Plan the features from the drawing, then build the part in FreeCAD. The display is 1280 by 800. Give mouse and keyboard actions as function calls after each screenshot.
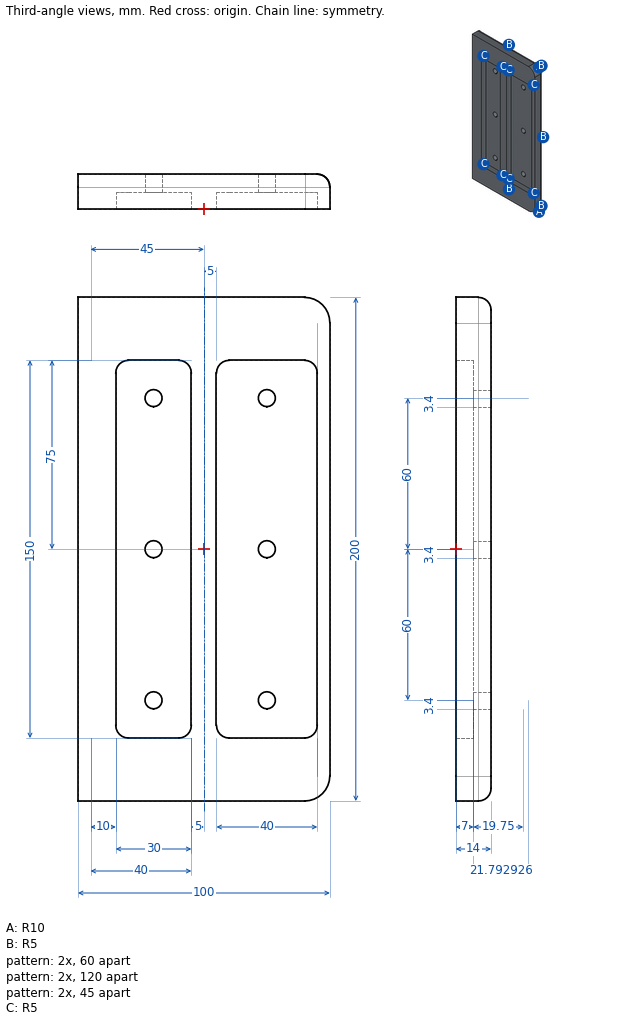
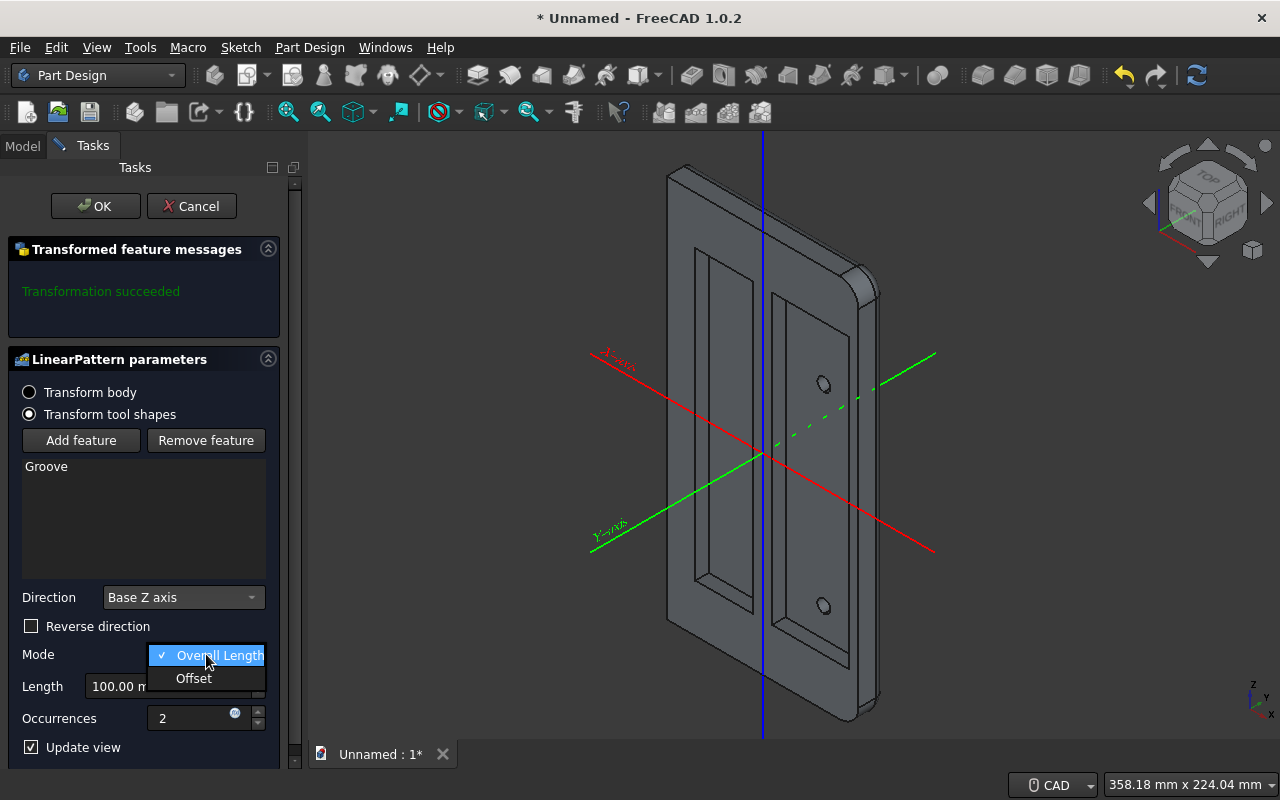
click(206, 678)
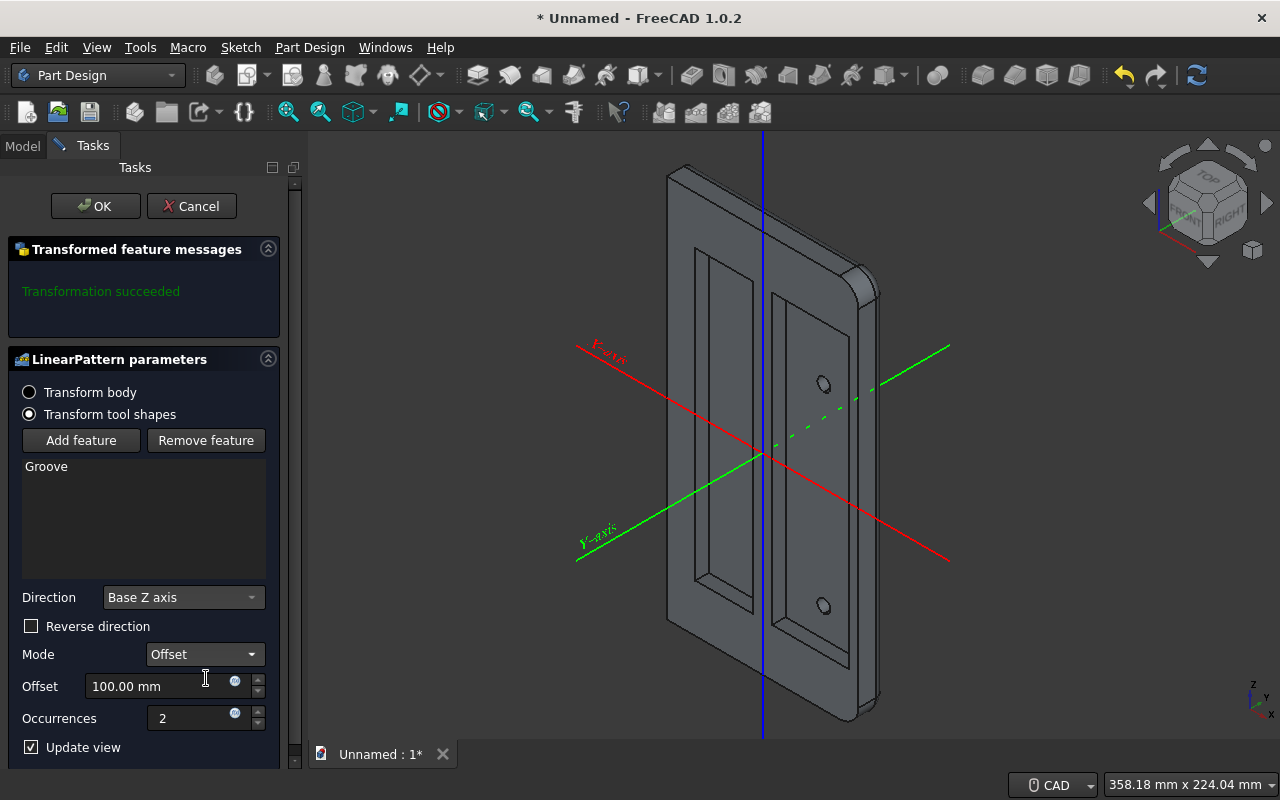
triple_click(168, 686)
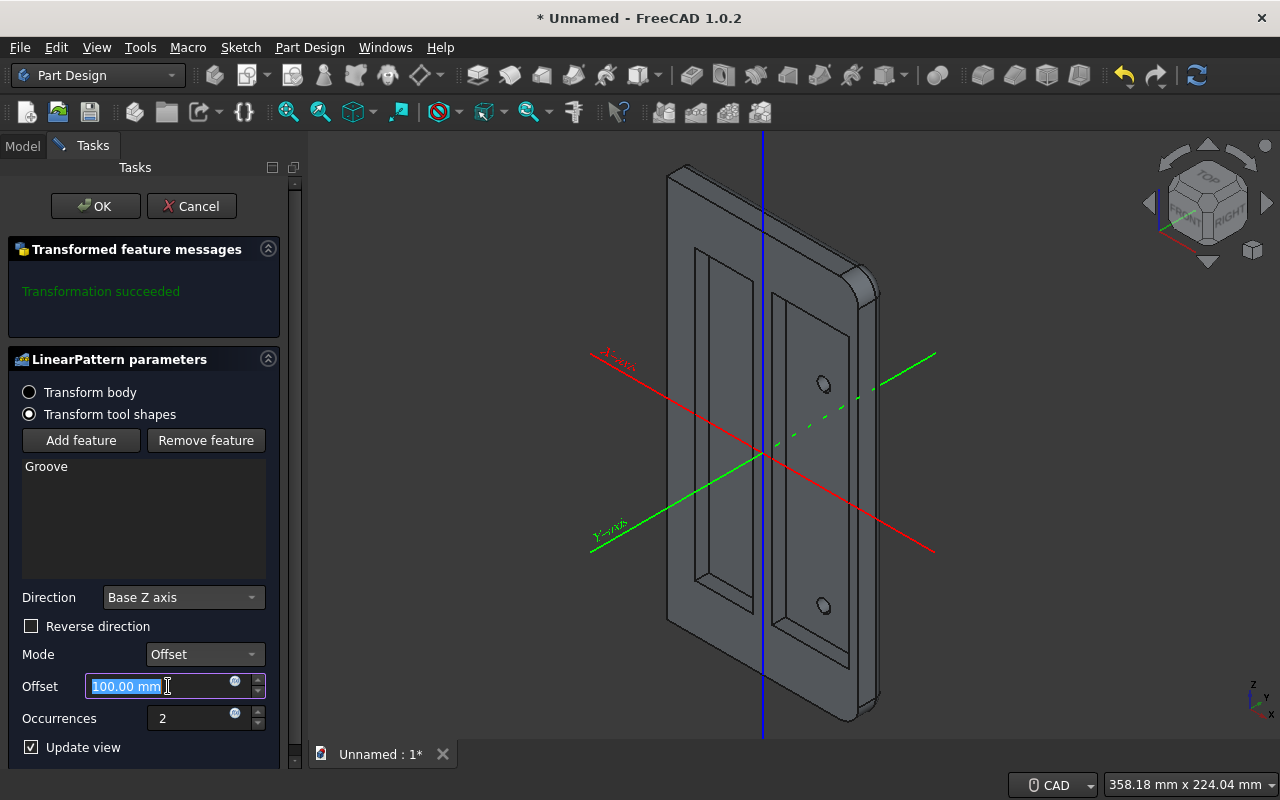
text(60)
key(Tab)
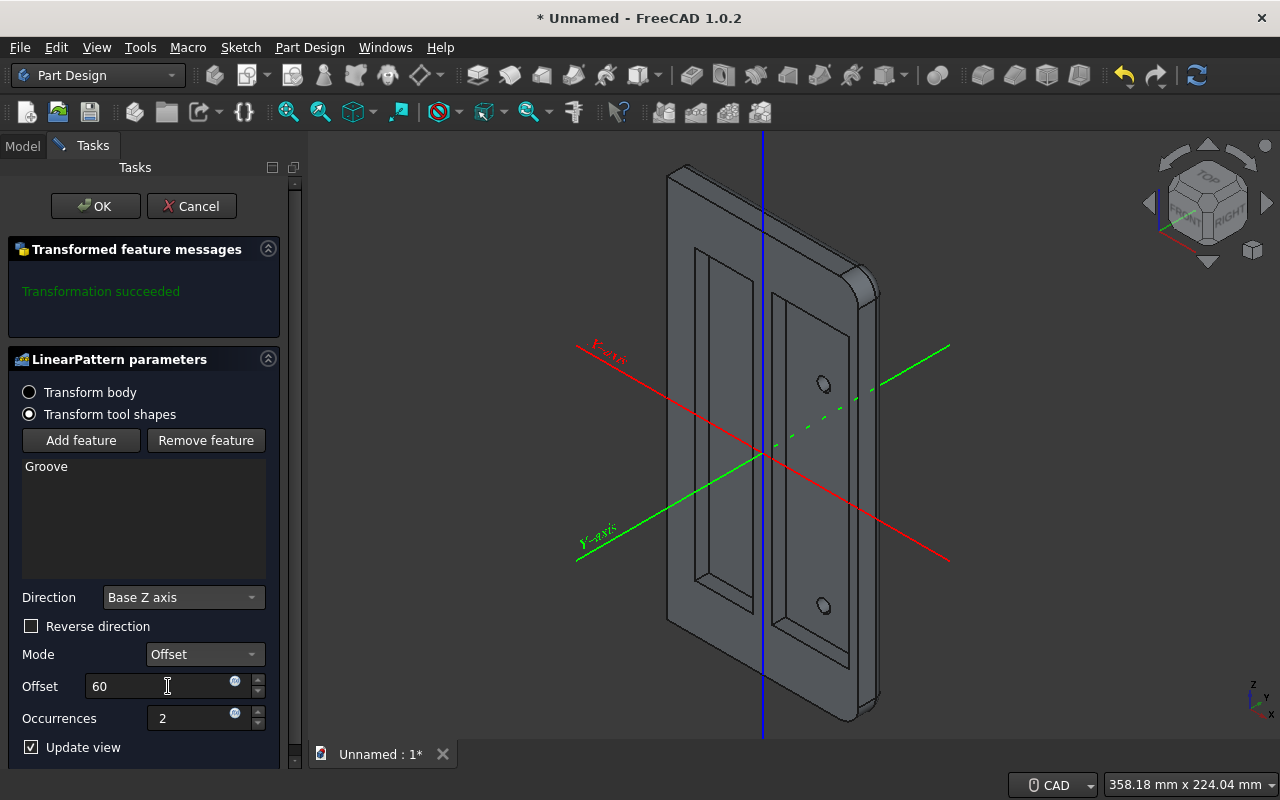
triple_click(198, 718)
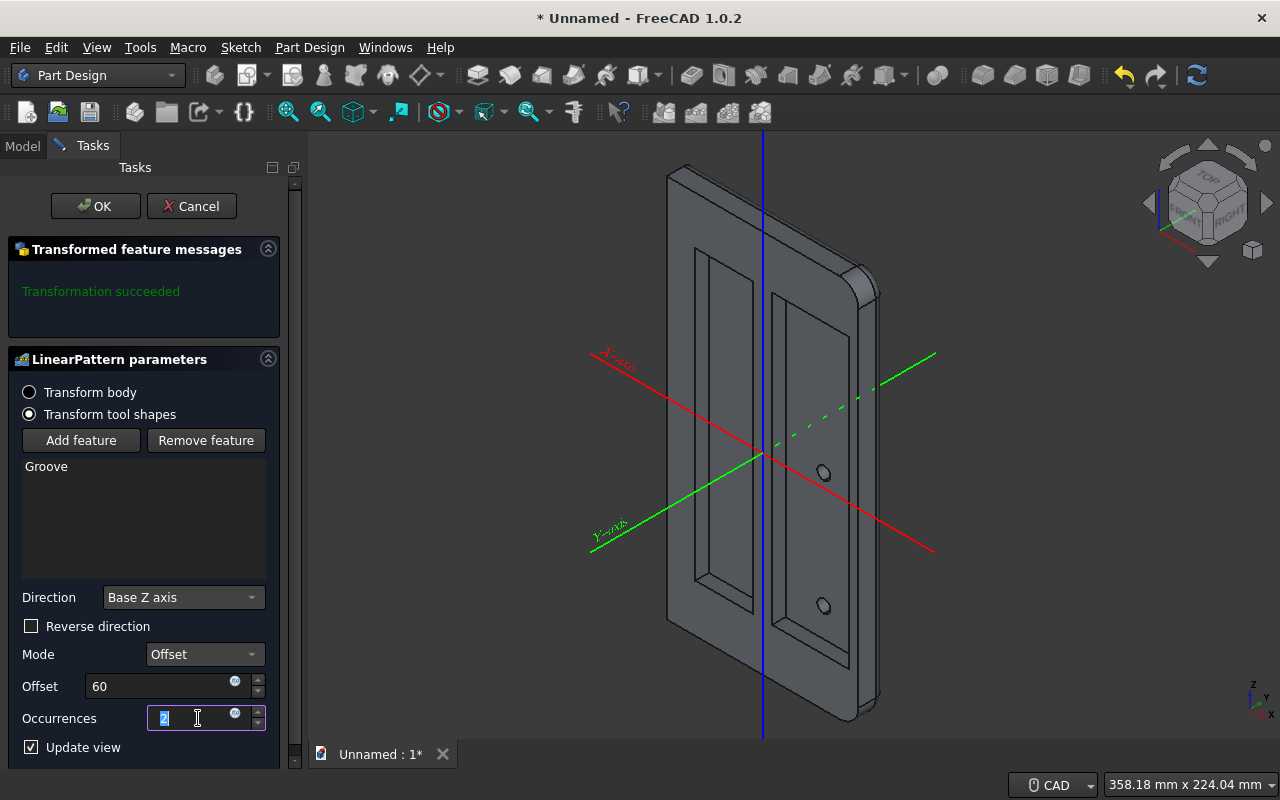
text(2)
key(Tab)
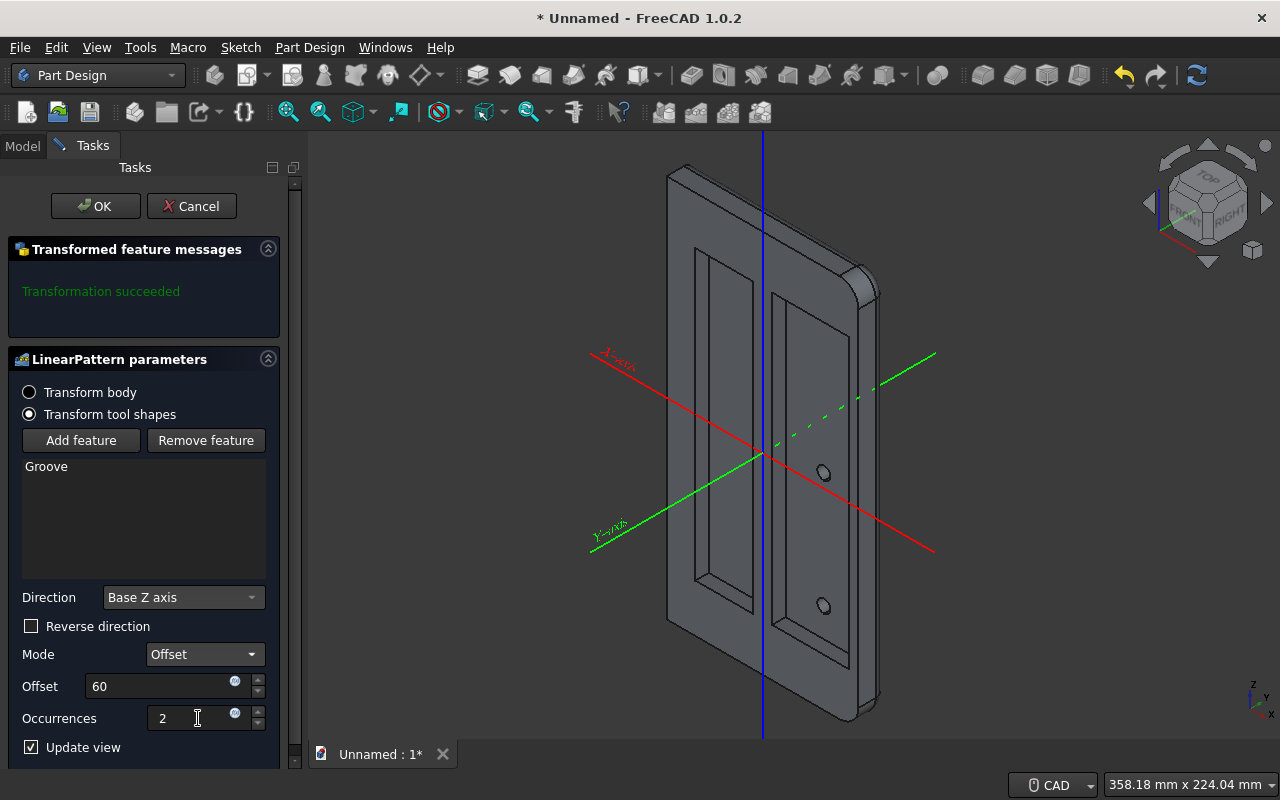
click(96, 206)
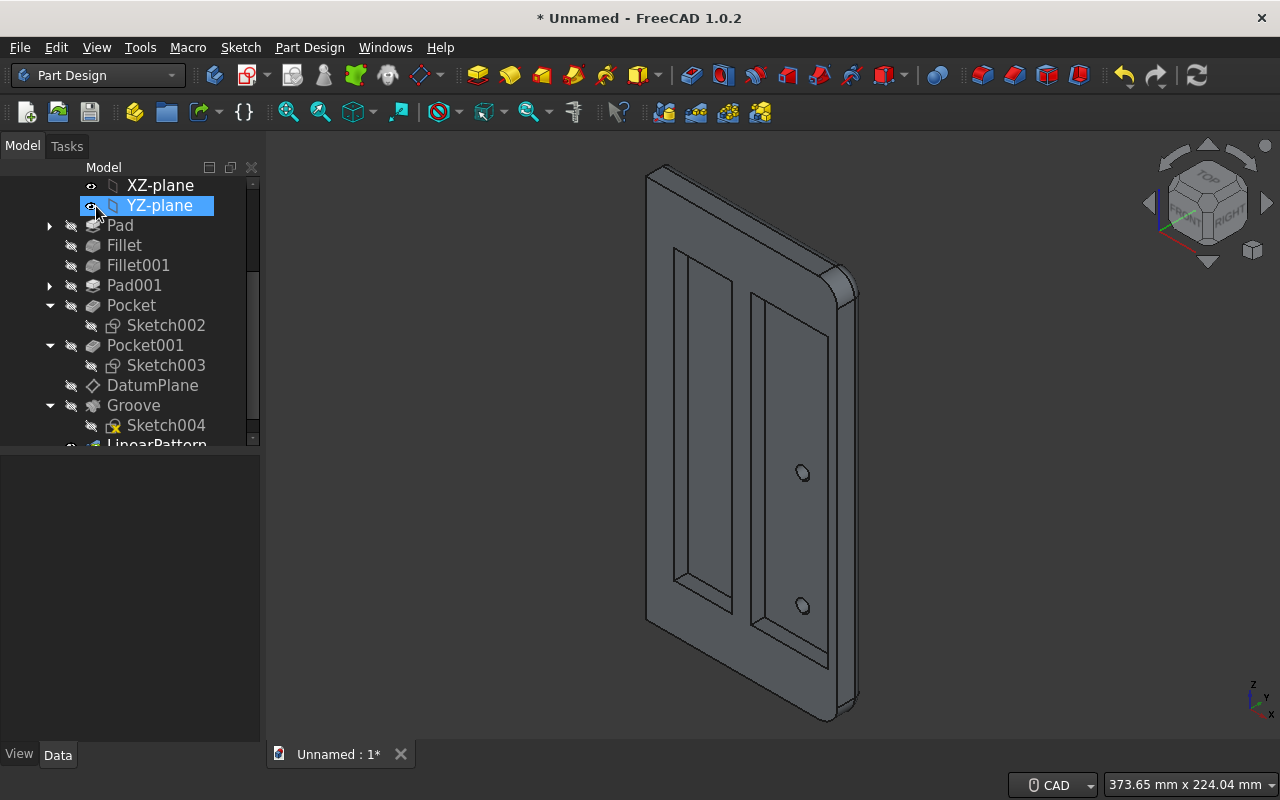
click(116, 406)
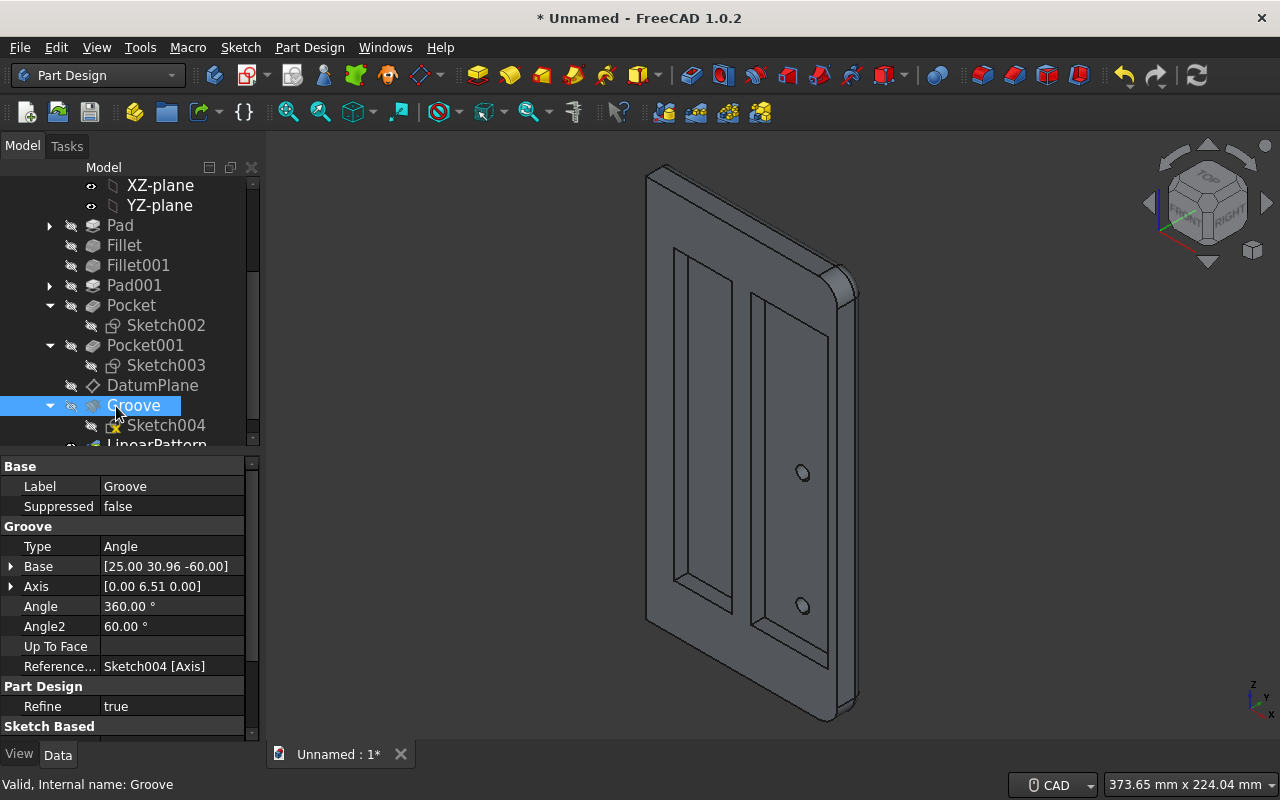
click(696, 112)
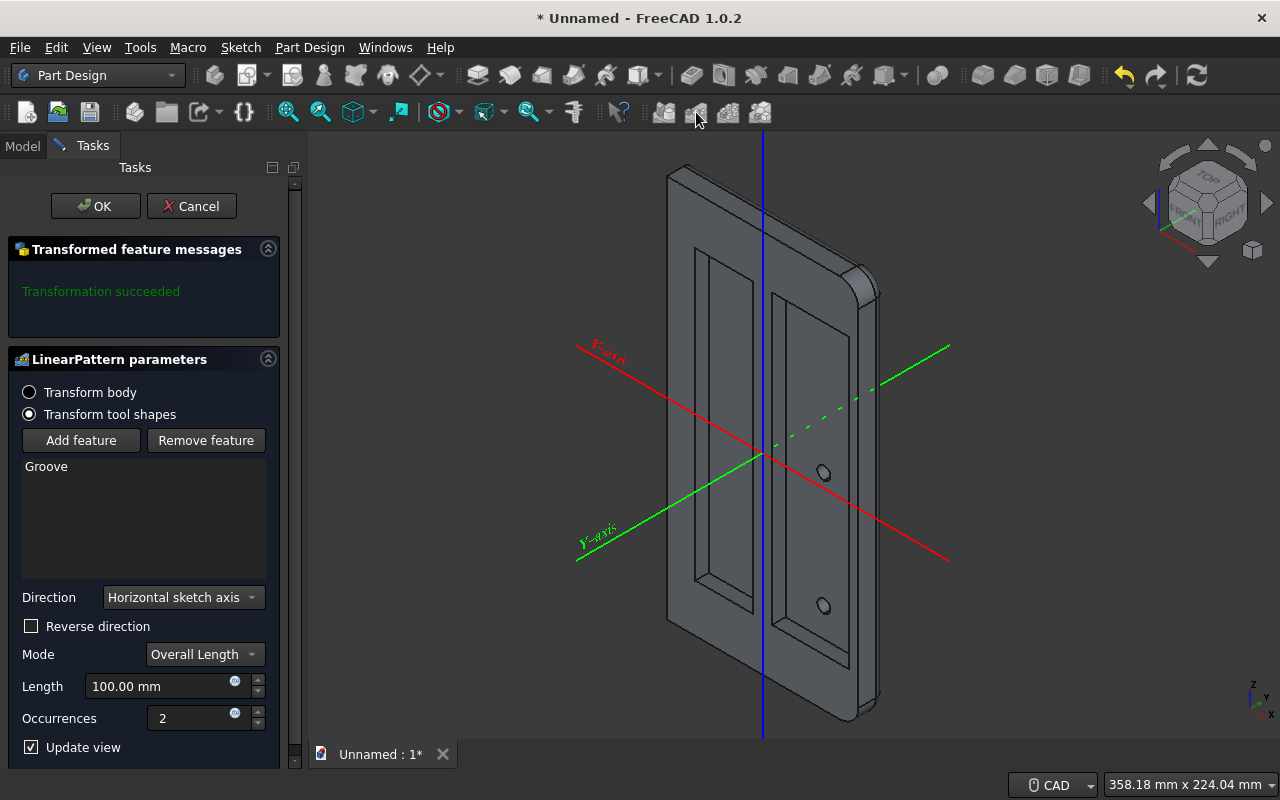
click(184, 598)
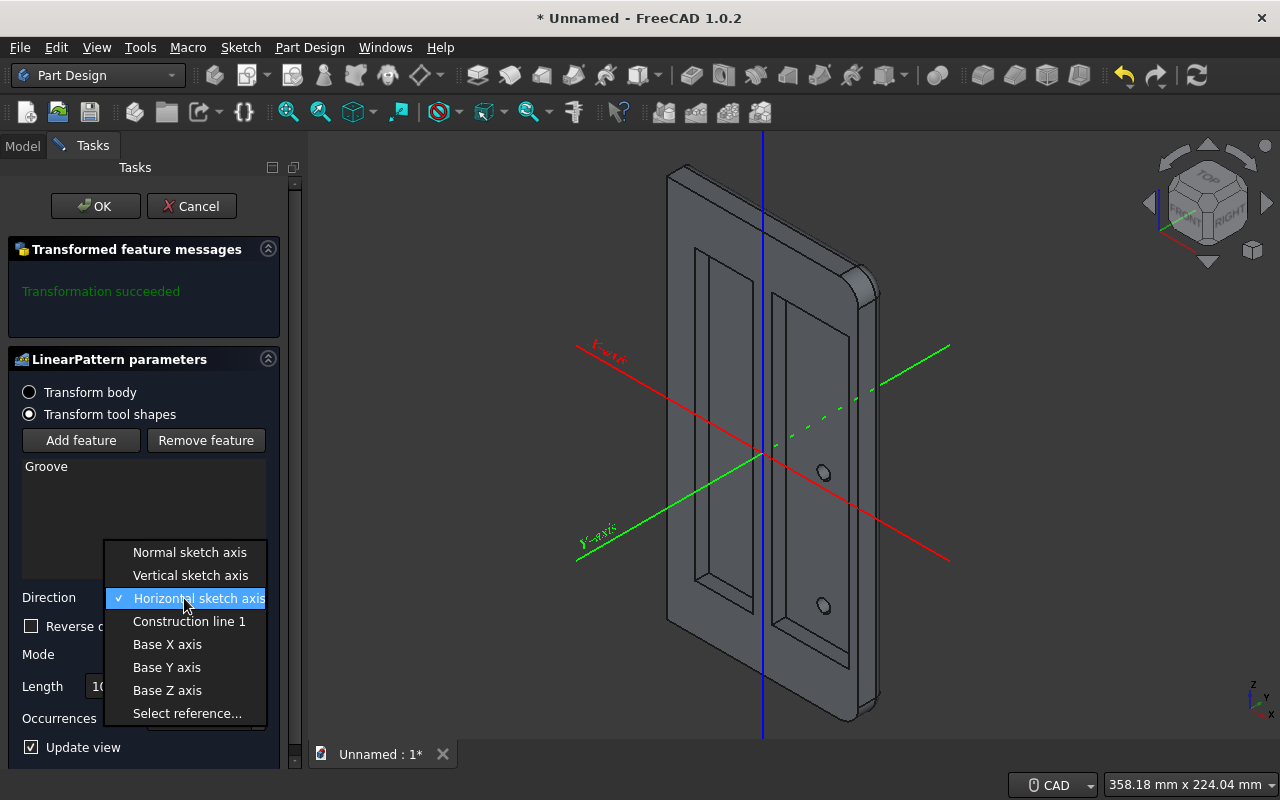
click(184, 690)